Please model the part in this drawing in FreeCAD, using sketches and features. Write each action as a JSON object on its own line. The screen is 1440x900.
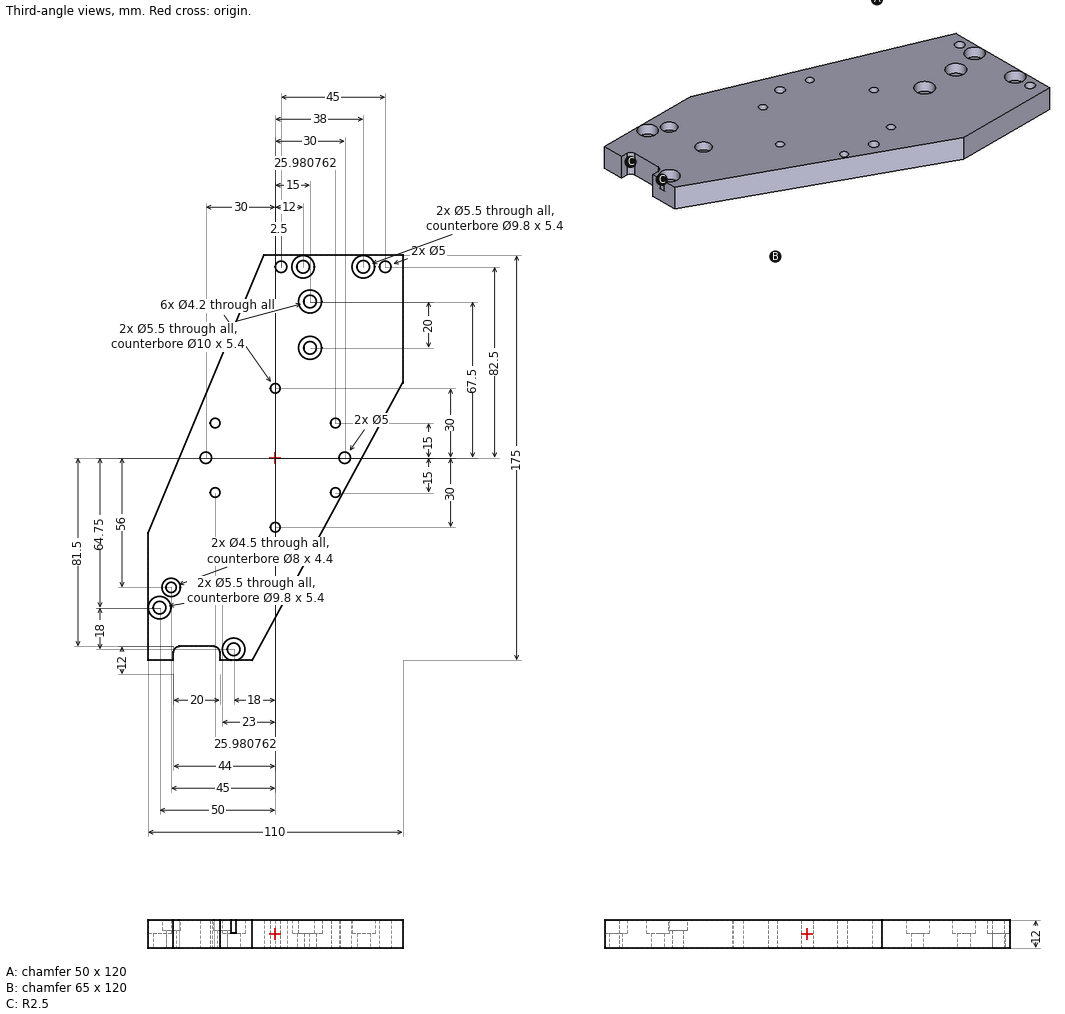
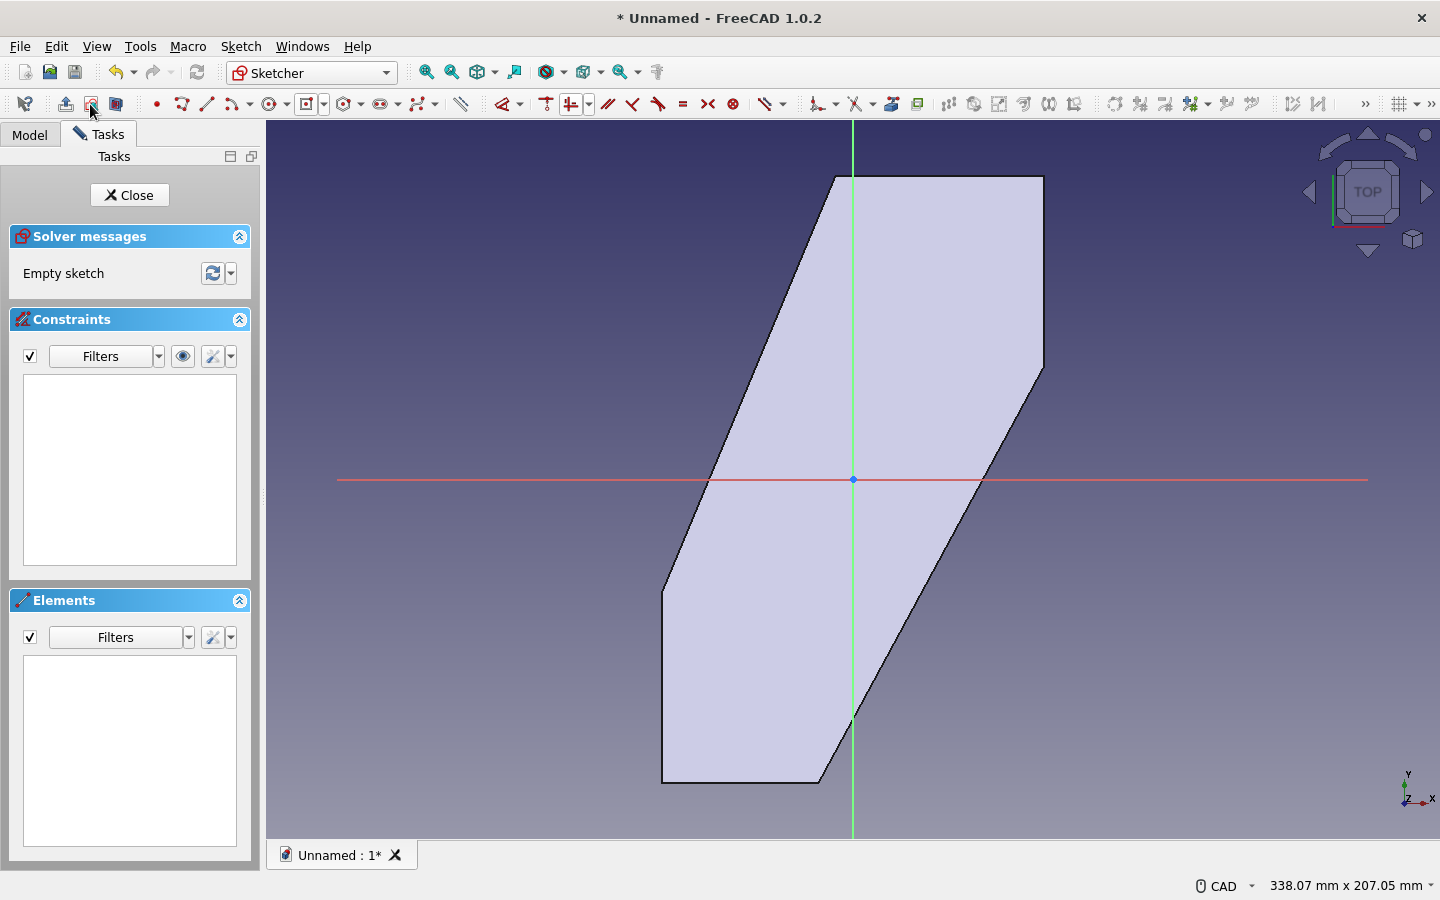
{"action": "scroll", "coordinate": [1256, 148], "scroll_direction": "up", "scroll_amount": 2}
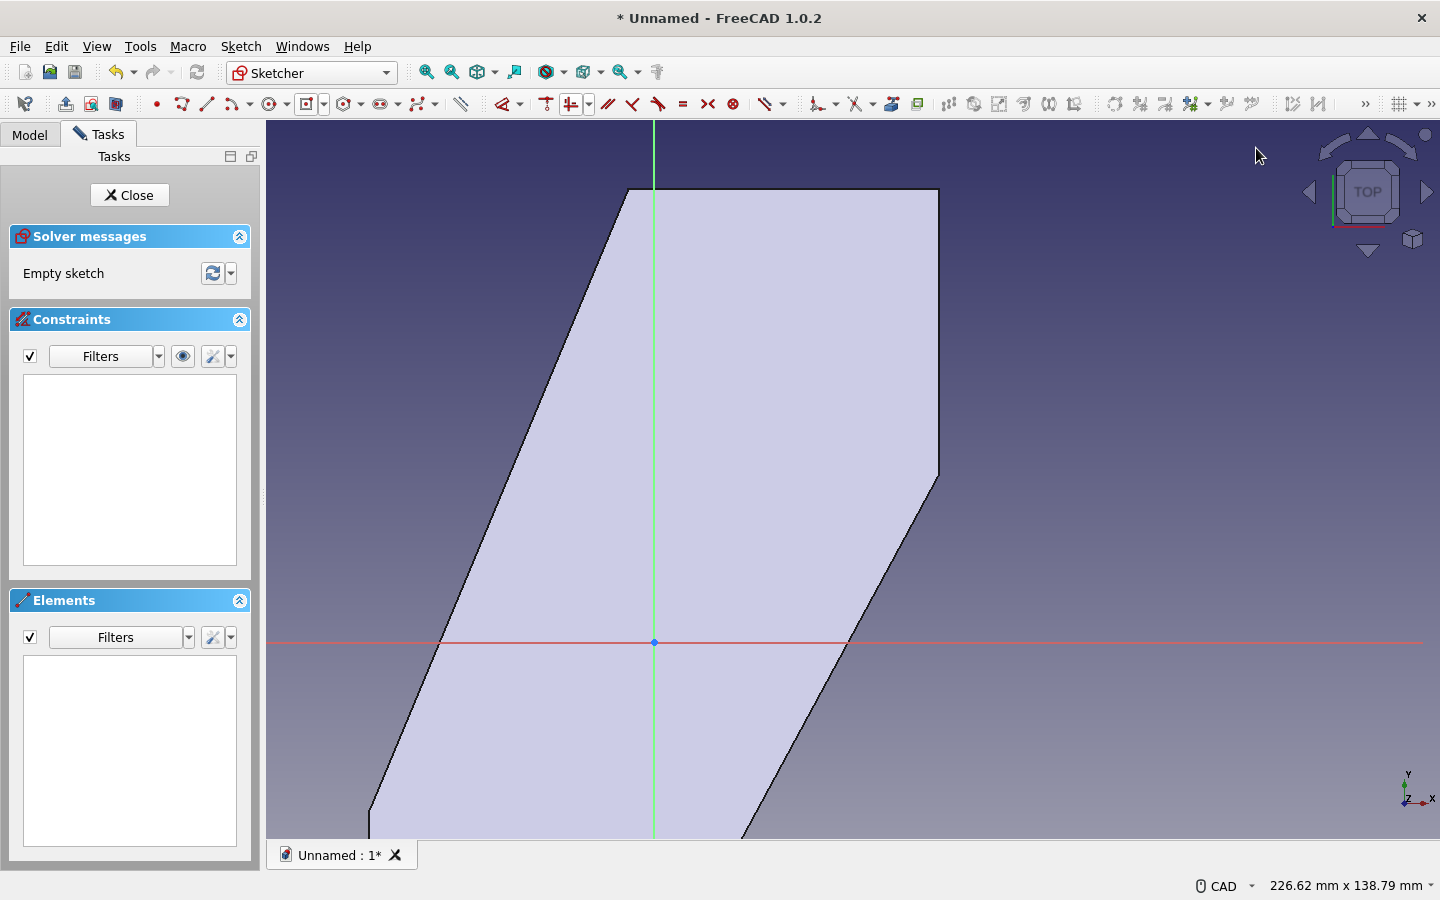
{"action": "left_click", "coordinate": [268, 104]}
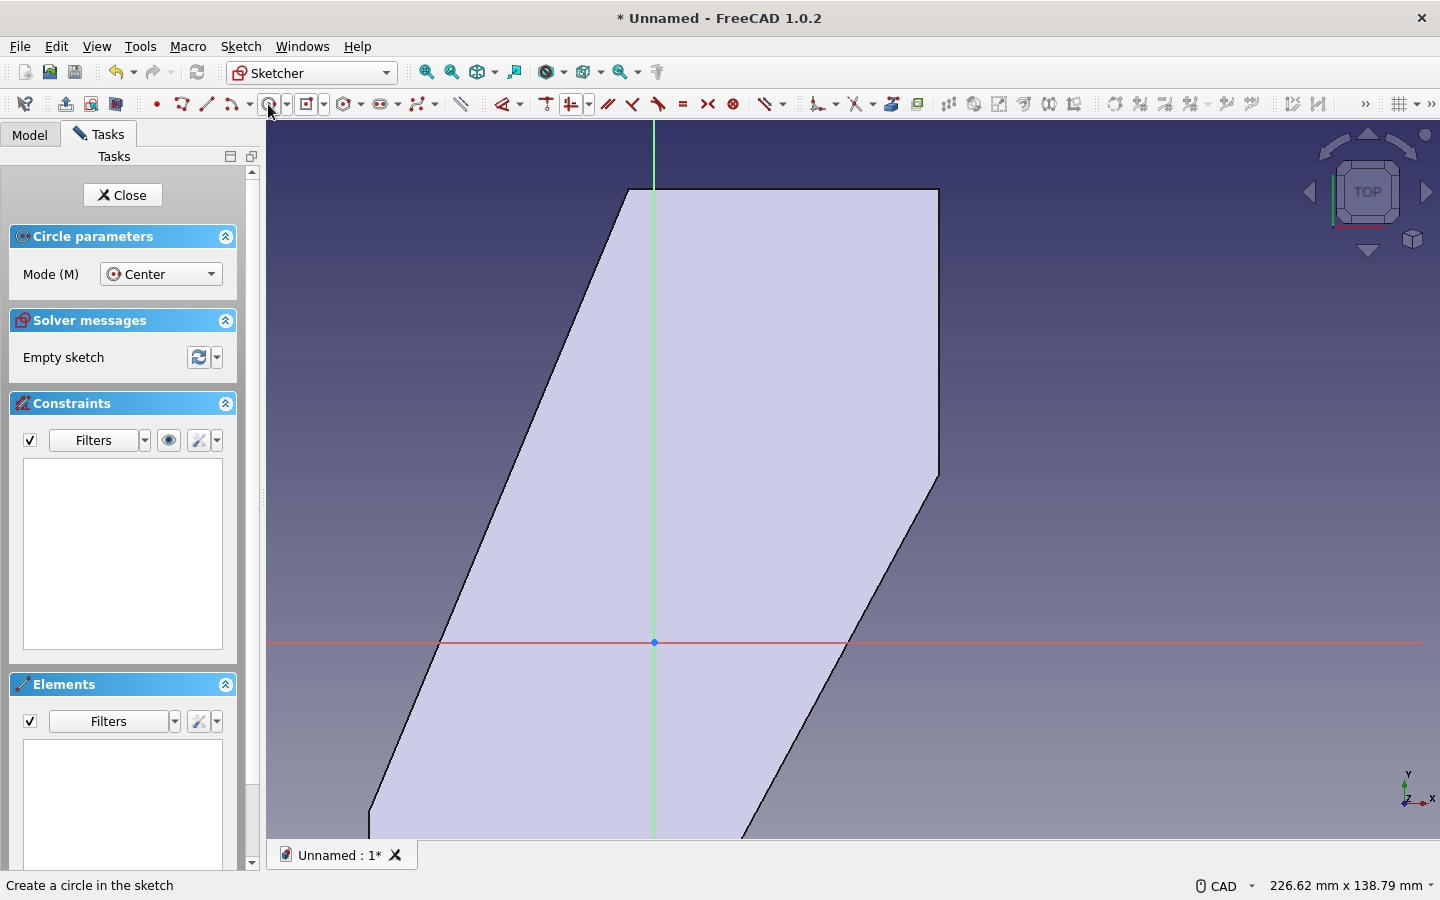
{"action": "scroll", "coordinate": [900, 215], "scroll_direction": "up", "scroll_amount": 3}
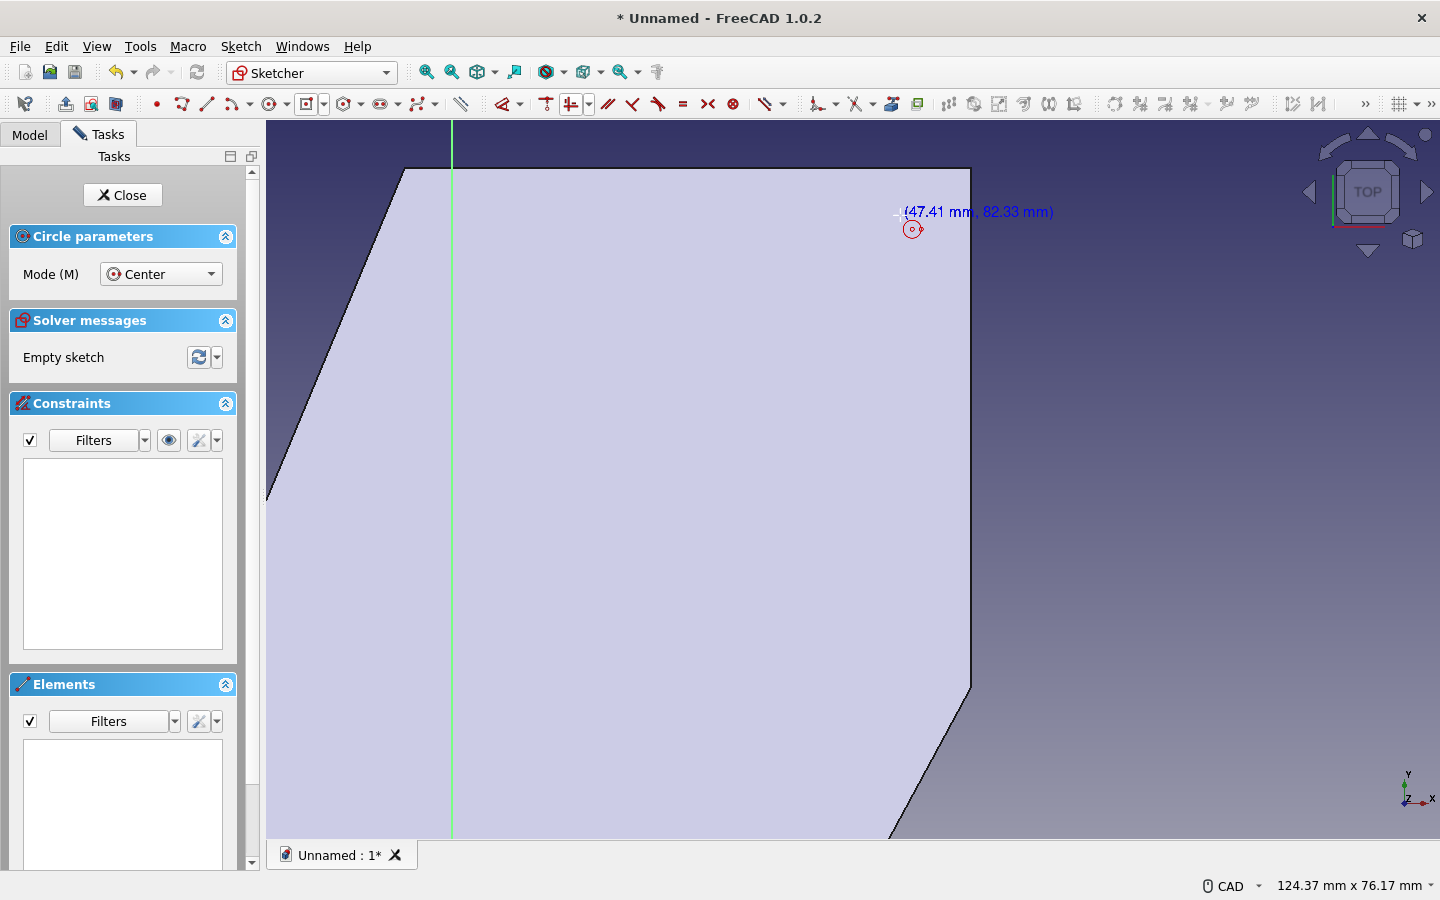
{"action": "left_click", "coordinate": [900, 215]}
{"action": "left_click", "coordinate": [917, 198]}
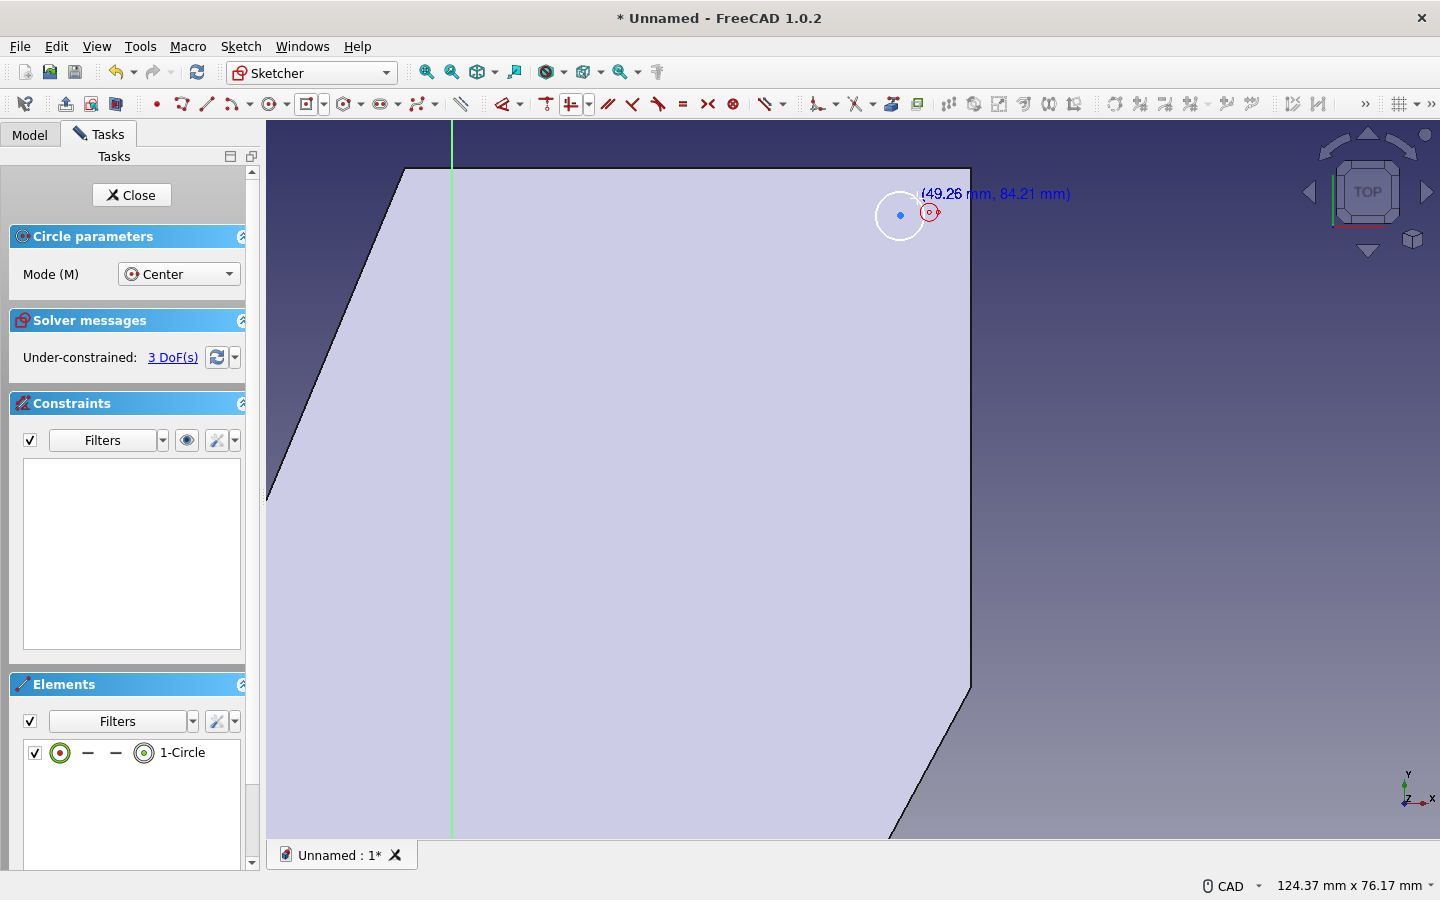
{"action": "left_click", "coordinate": [476, 215]}
{"action": "left_click", "coordinate": [492, 198]}
{"action": "key", "text": "Escape"}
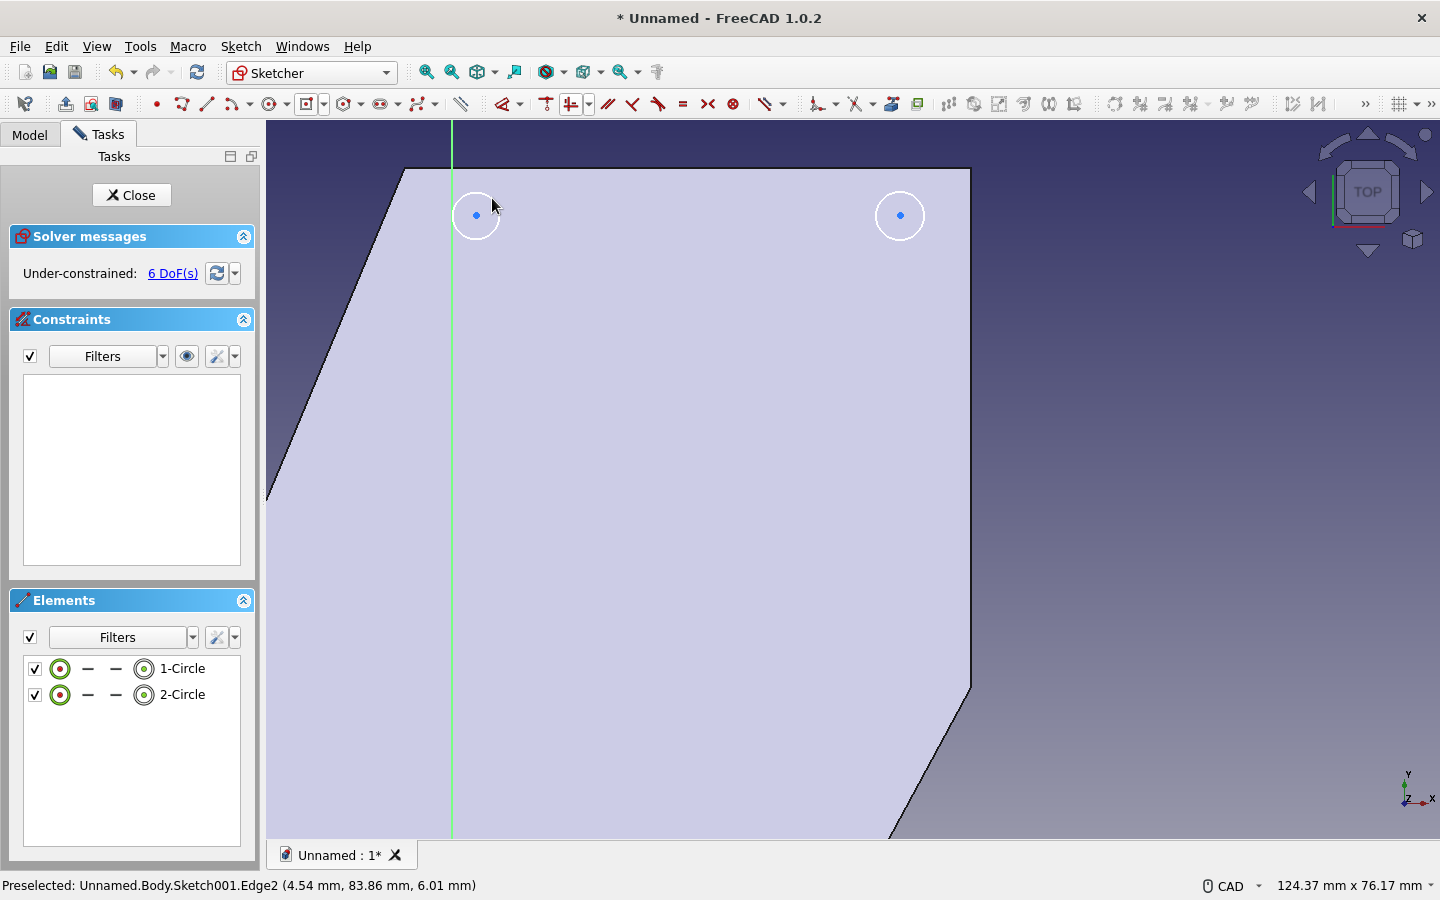
{"action": "left_click", "coordinate": [917, 199]}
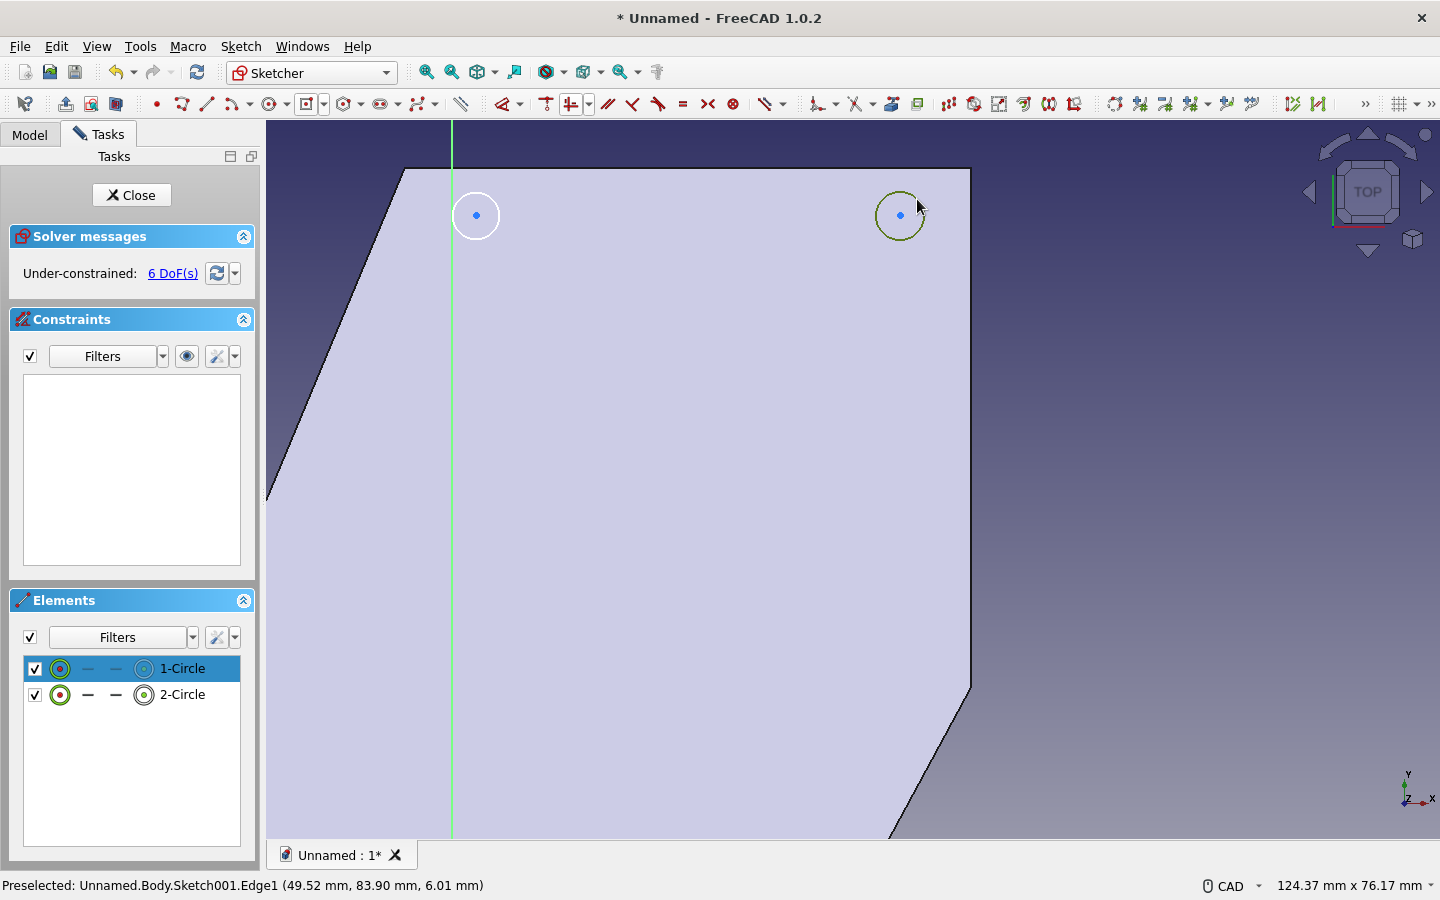
{"action": "left_click", "coordinate": [492, 199]}